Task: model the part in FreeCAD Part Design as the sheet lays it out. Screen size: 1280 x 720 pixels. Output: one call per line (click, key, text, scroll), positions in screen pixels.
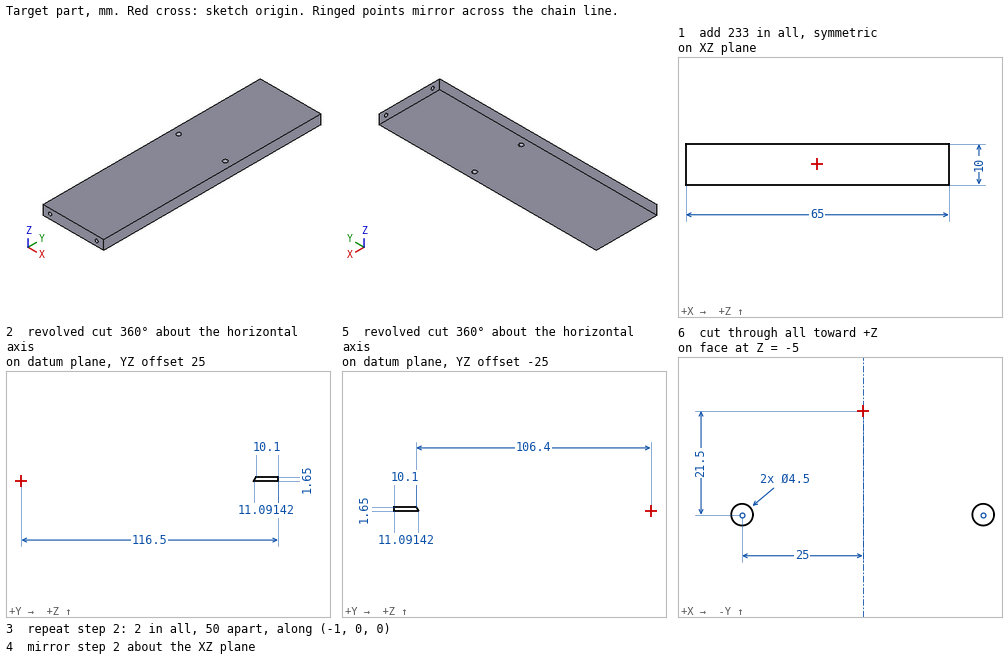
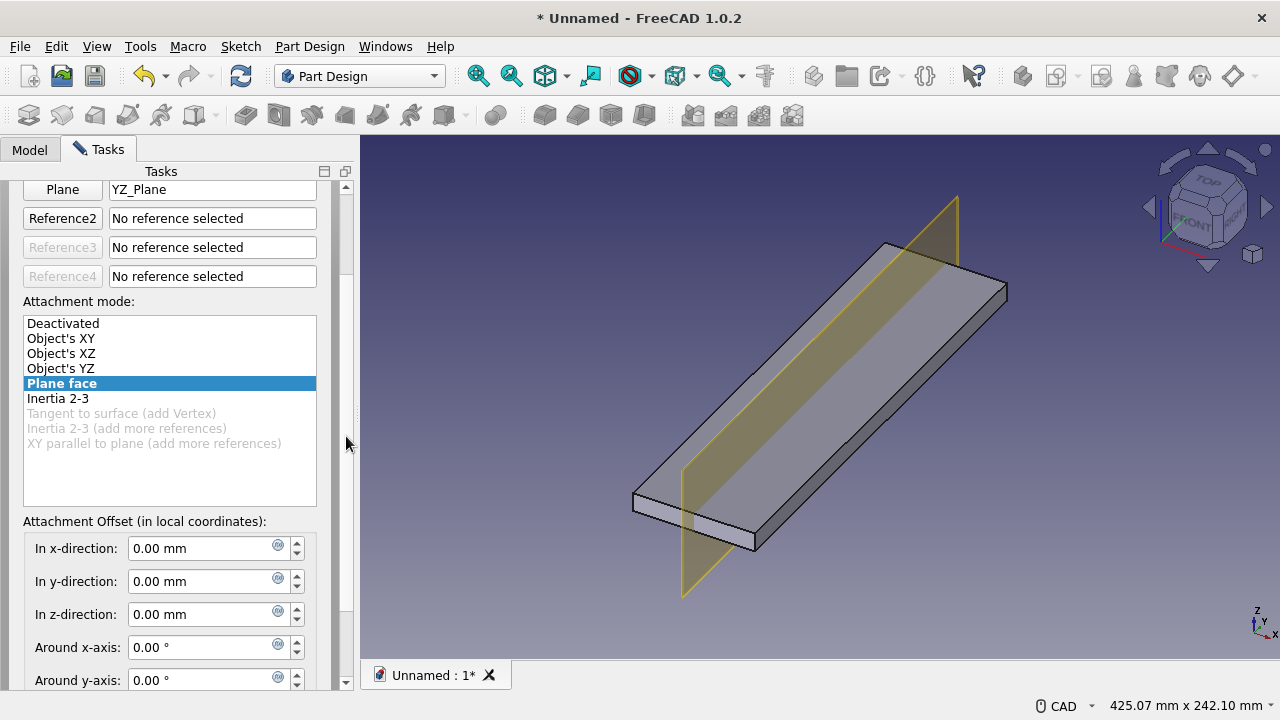
triple_click(210, 614)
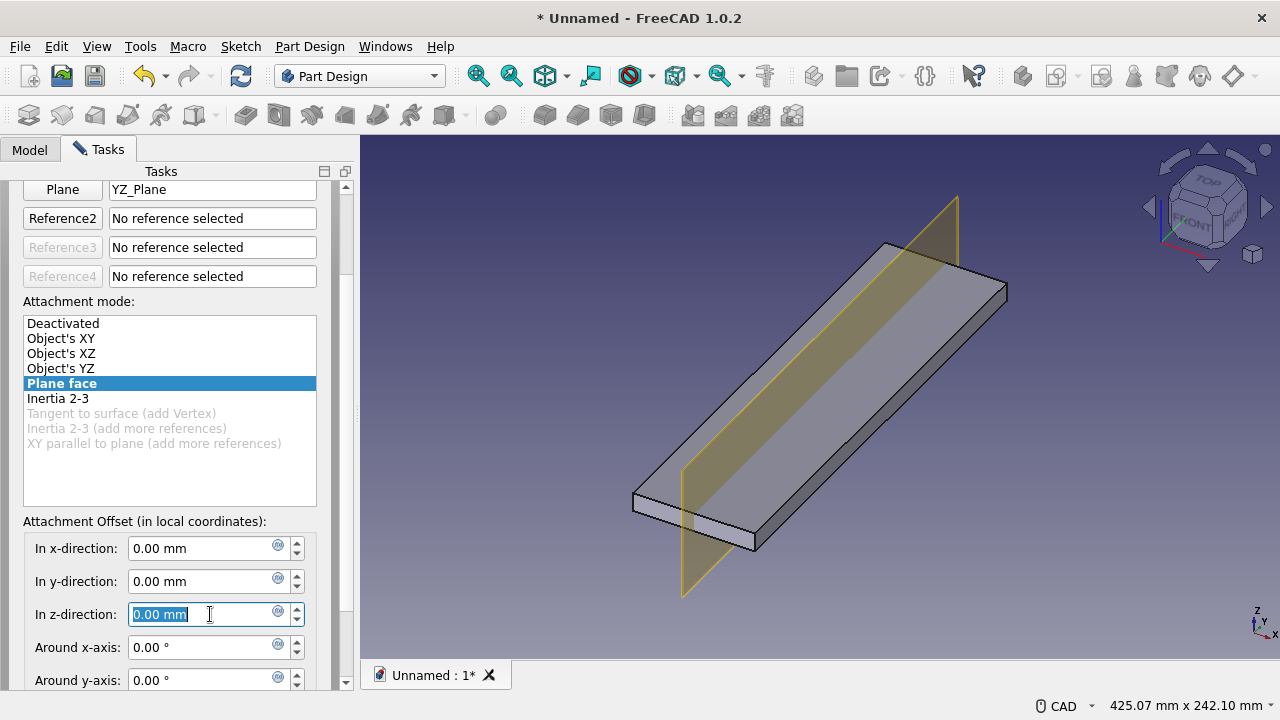
text(25)
key(Tab)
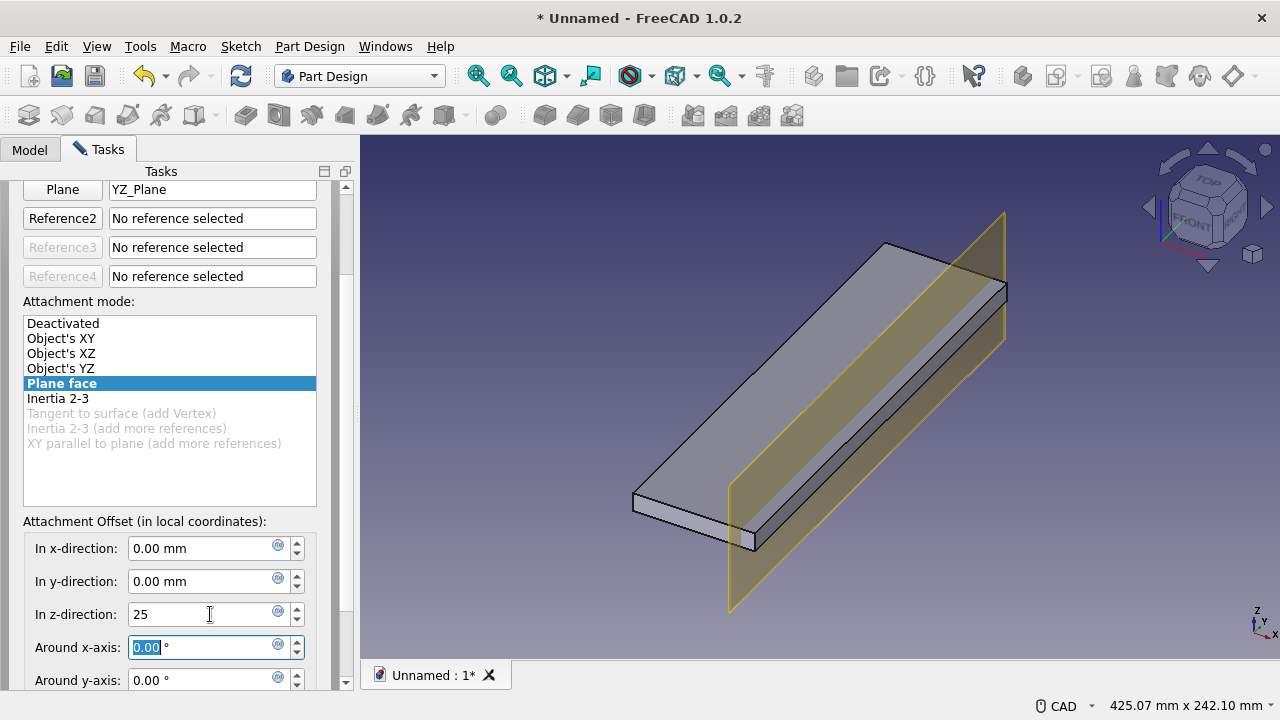
scroll(346, 436, up, 3)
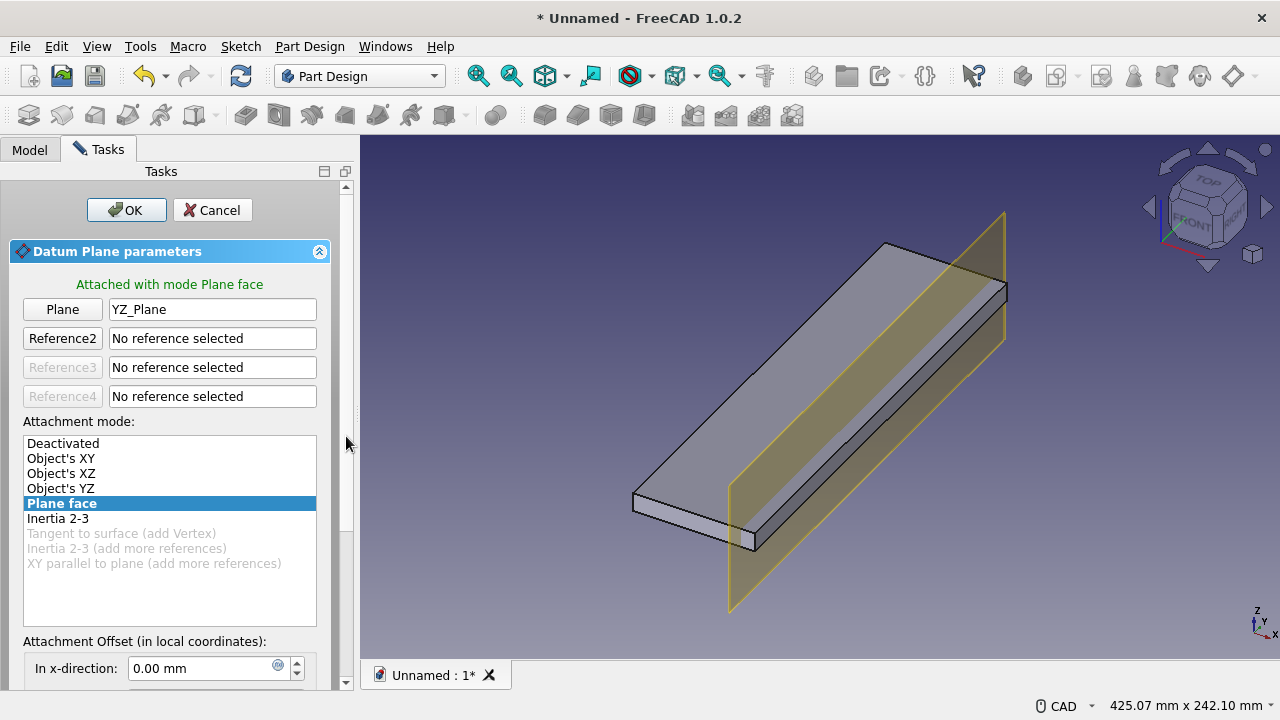
click(127, 210)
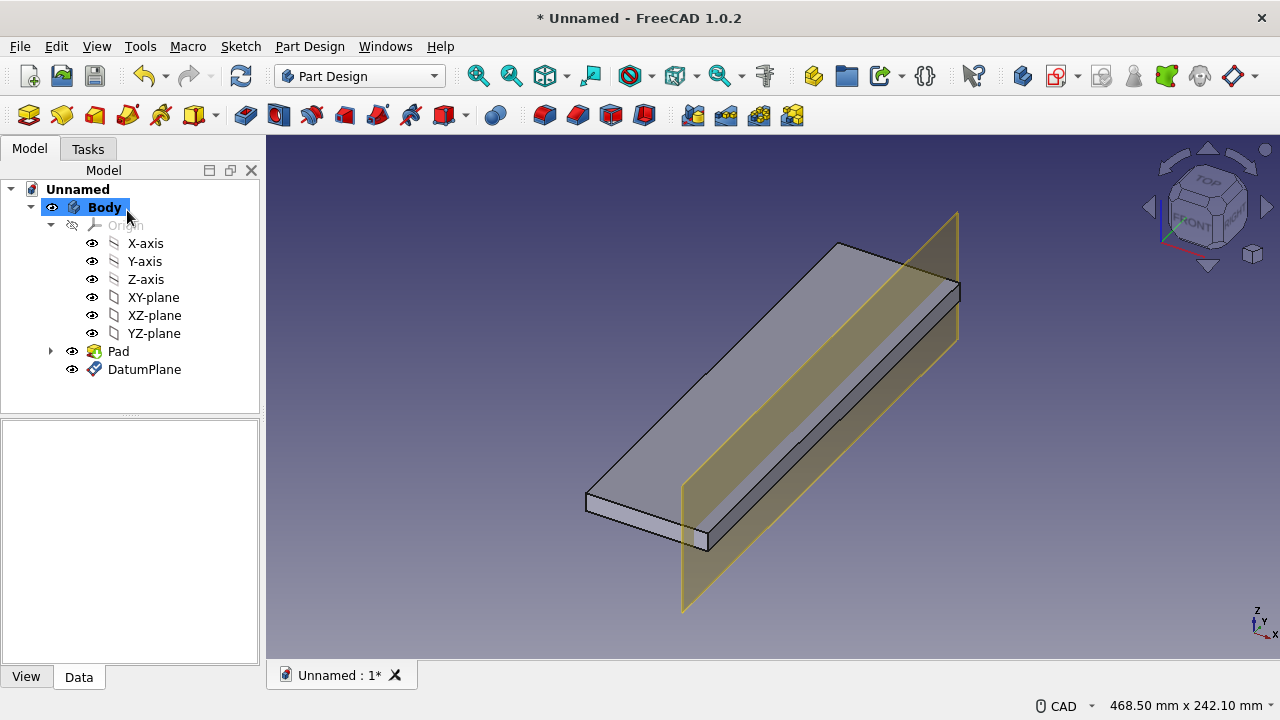
click(117, 369)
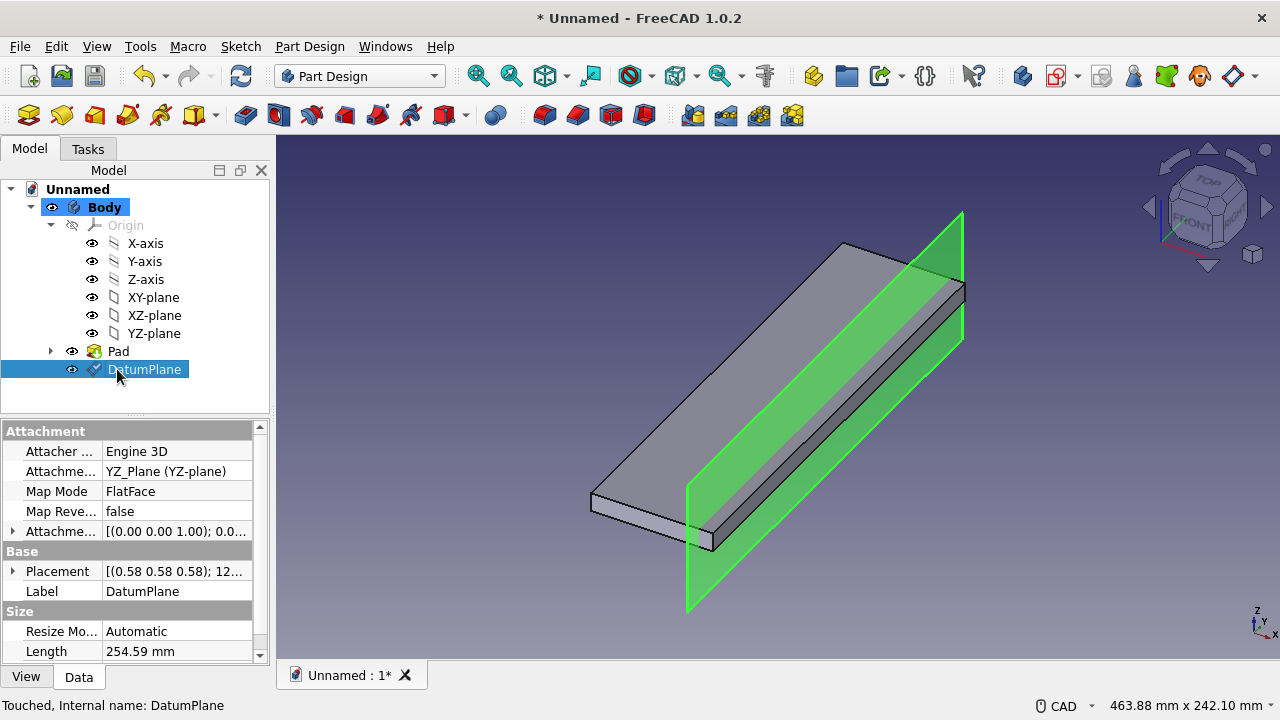
click(1056, 76)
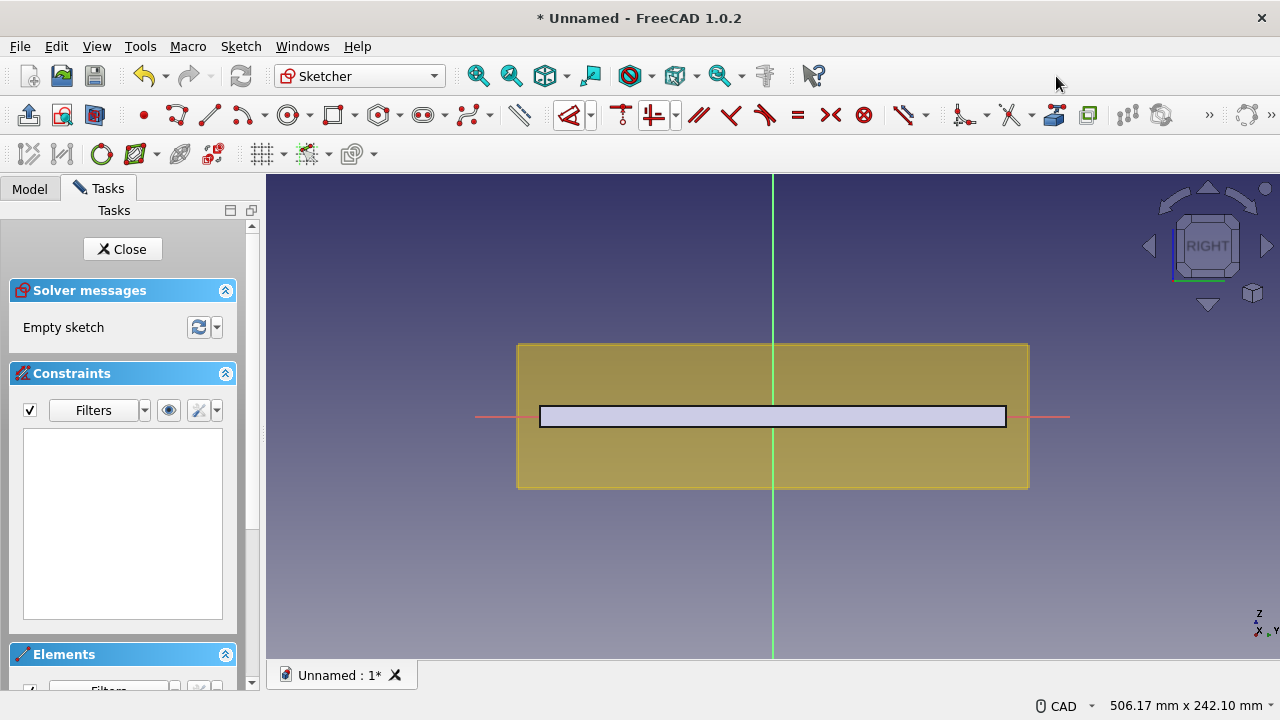
click(95, 116)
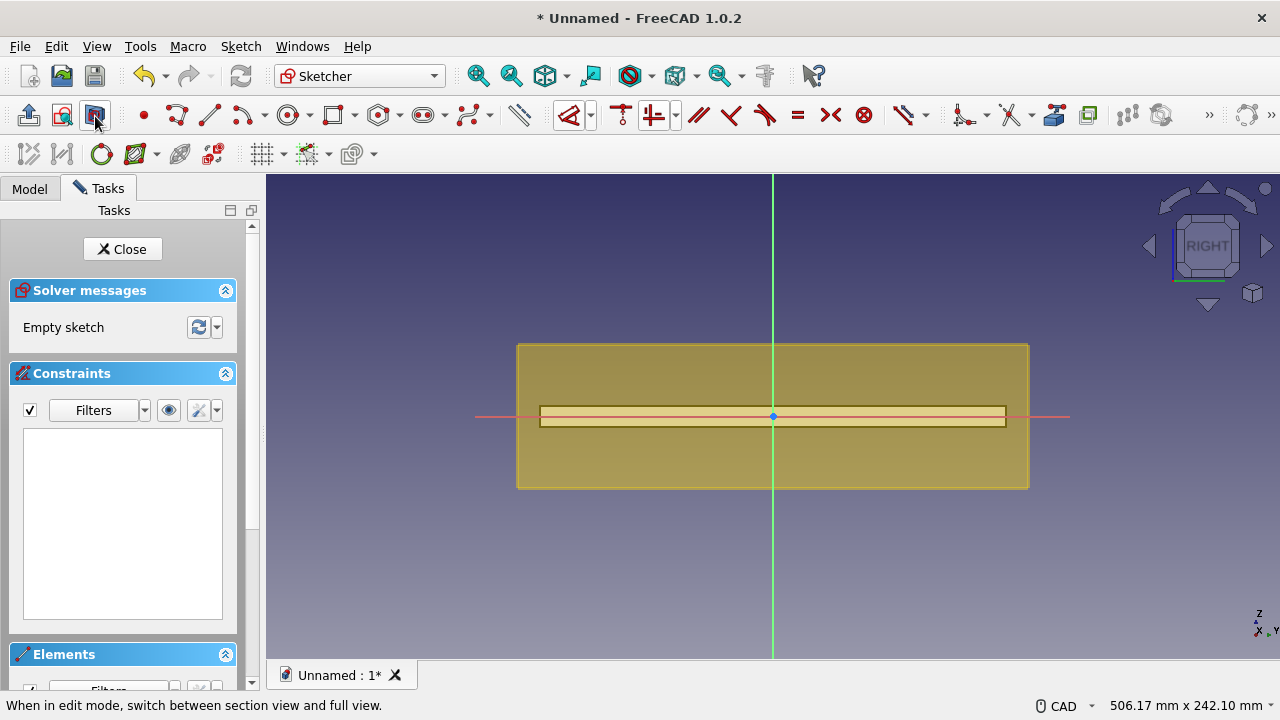
scroll(1011, 415, up, 15)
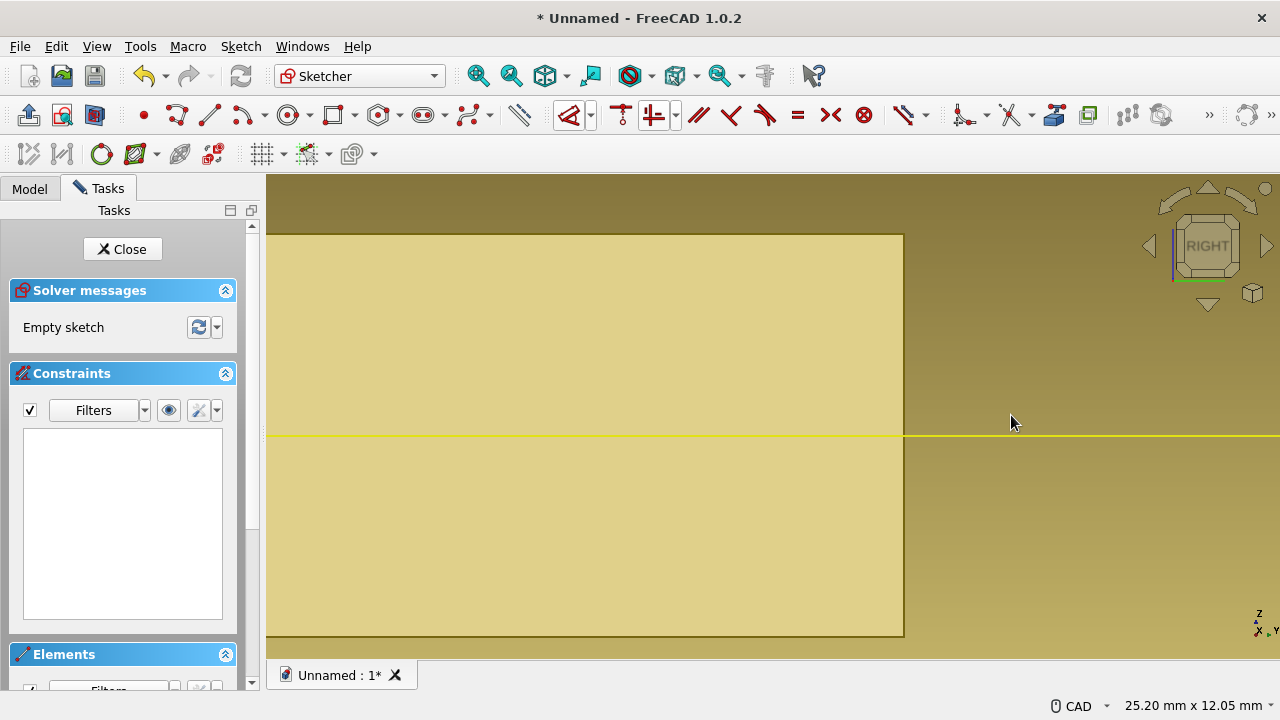
click(177, 116)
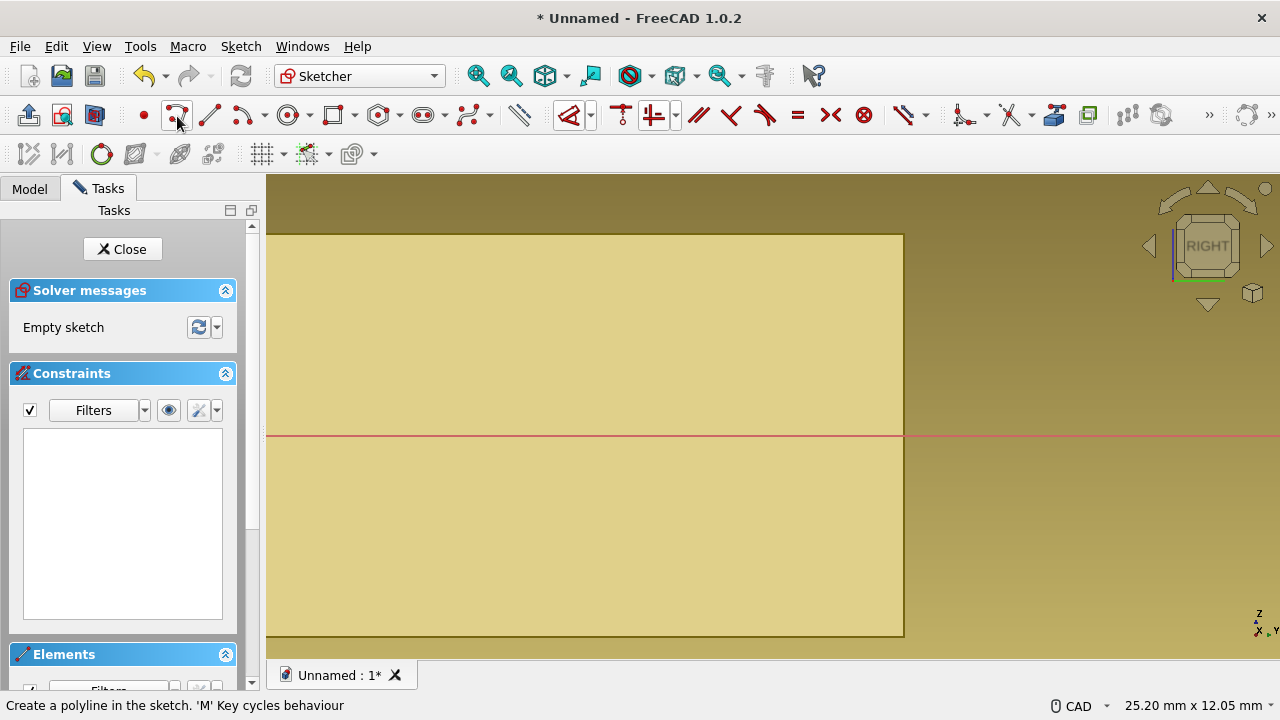
click(458, 436)
click(904, 427)
click(904, 369)
click(498, 369)
click(458, 436)
key(Escape)
key(Escape)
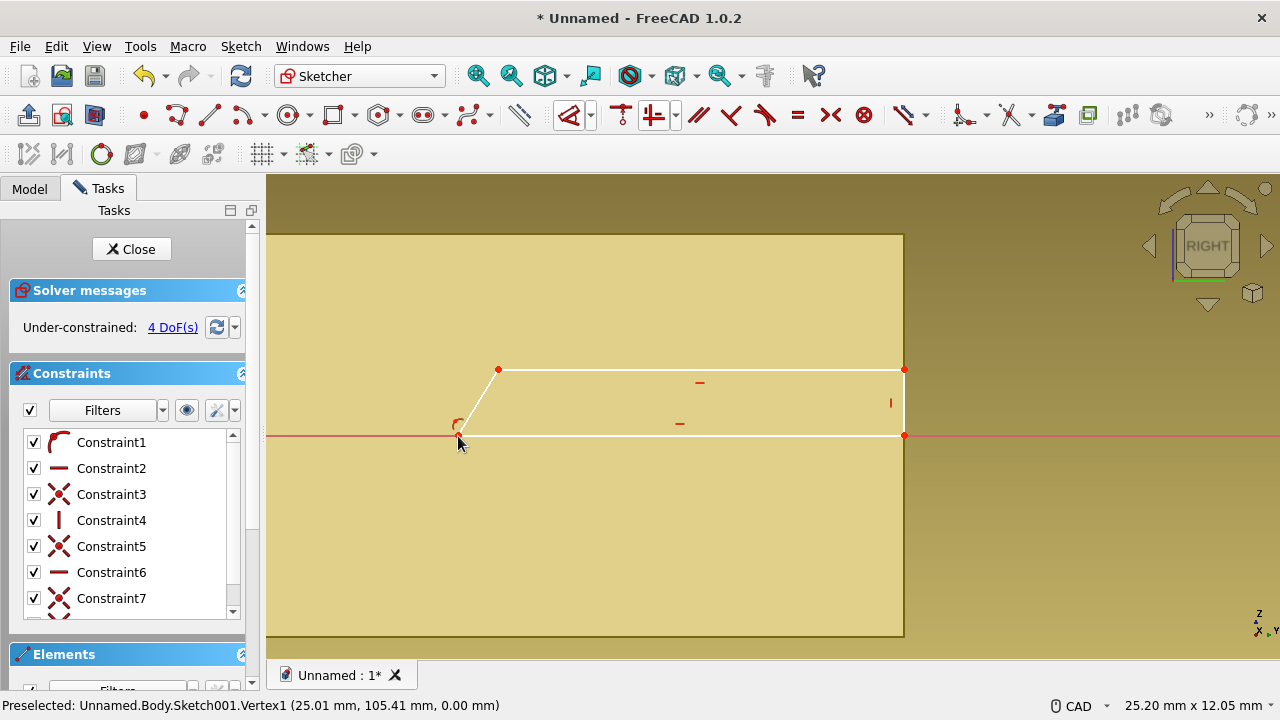
key(d)